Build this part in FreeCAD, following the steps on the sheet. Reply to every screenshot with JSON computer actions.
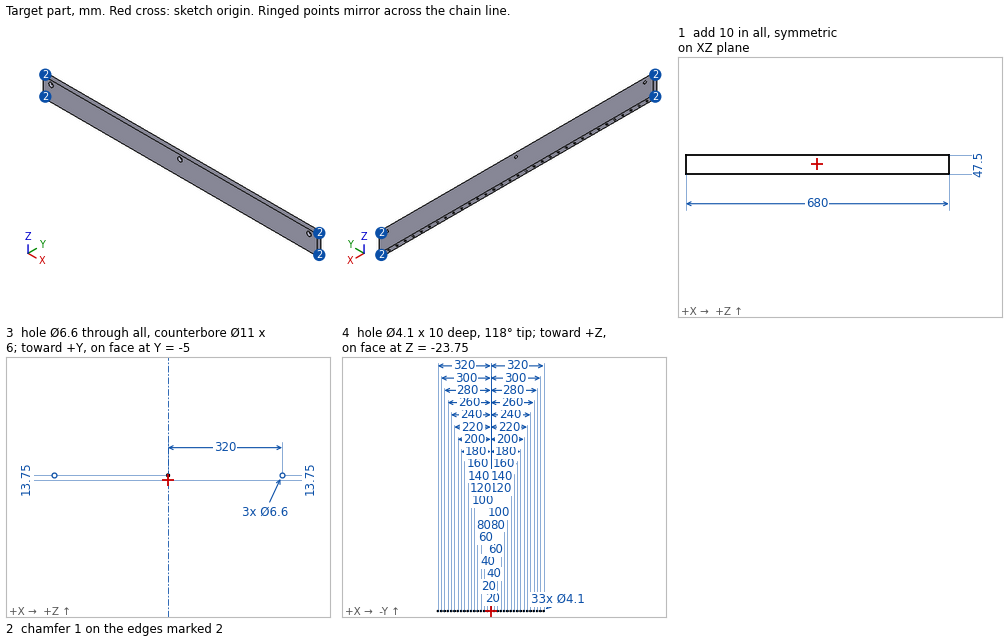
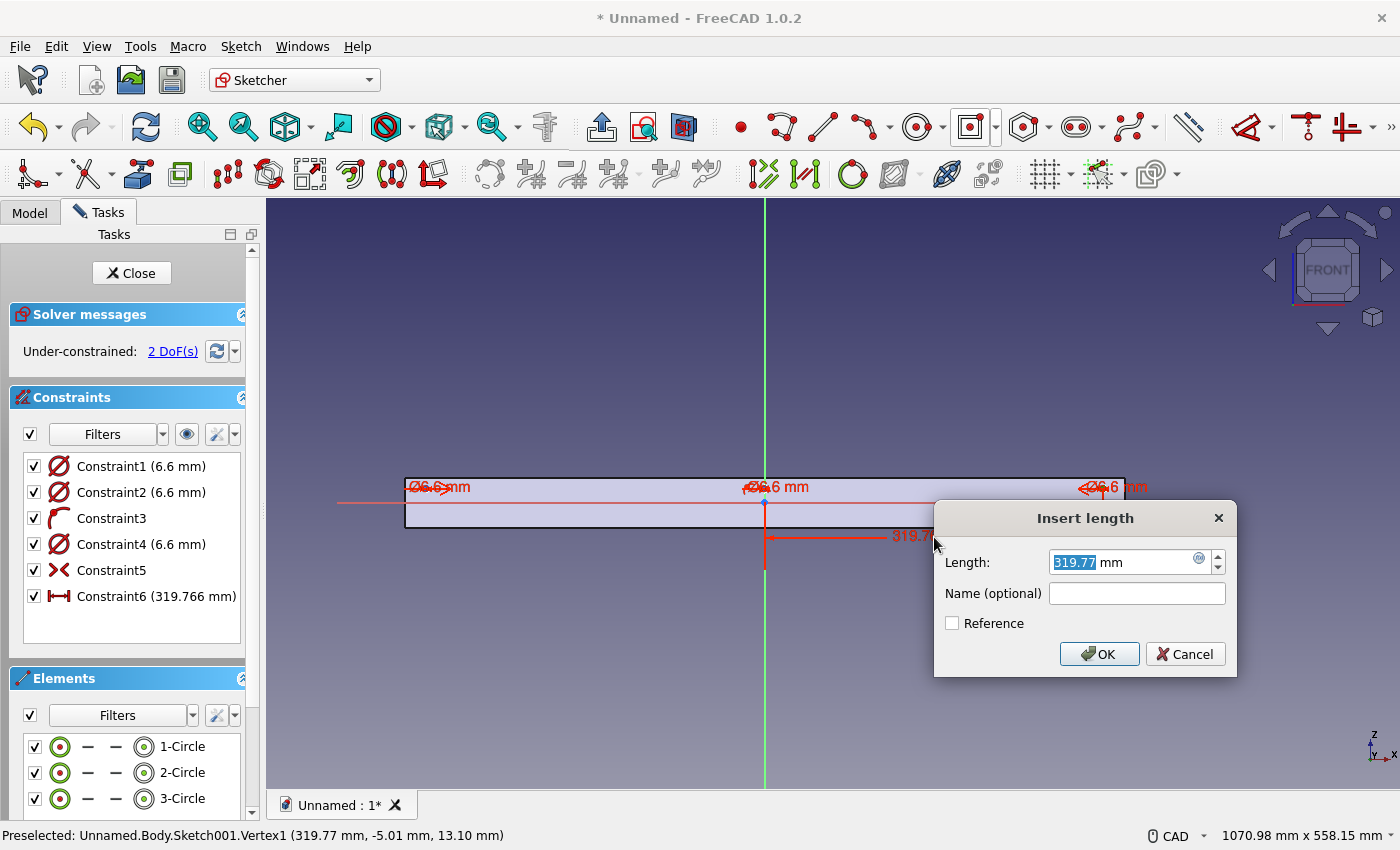
{"action": "type", "text": "320"}
{"action": "key", "text": "Return"}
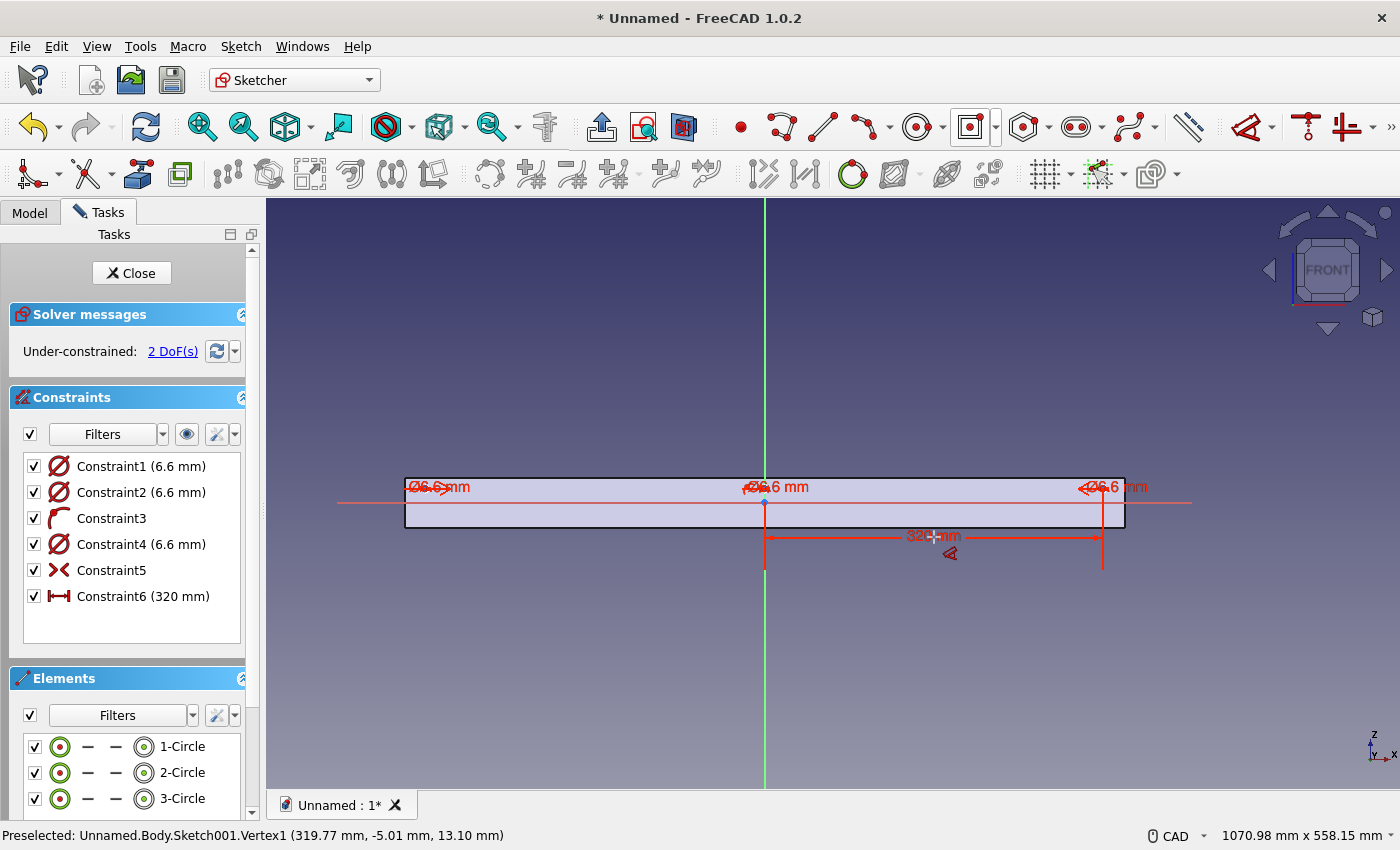
{"action": "scroll", "coordinate": [1103, 489], "scroll_direction": "up", "scroll_amount": 6}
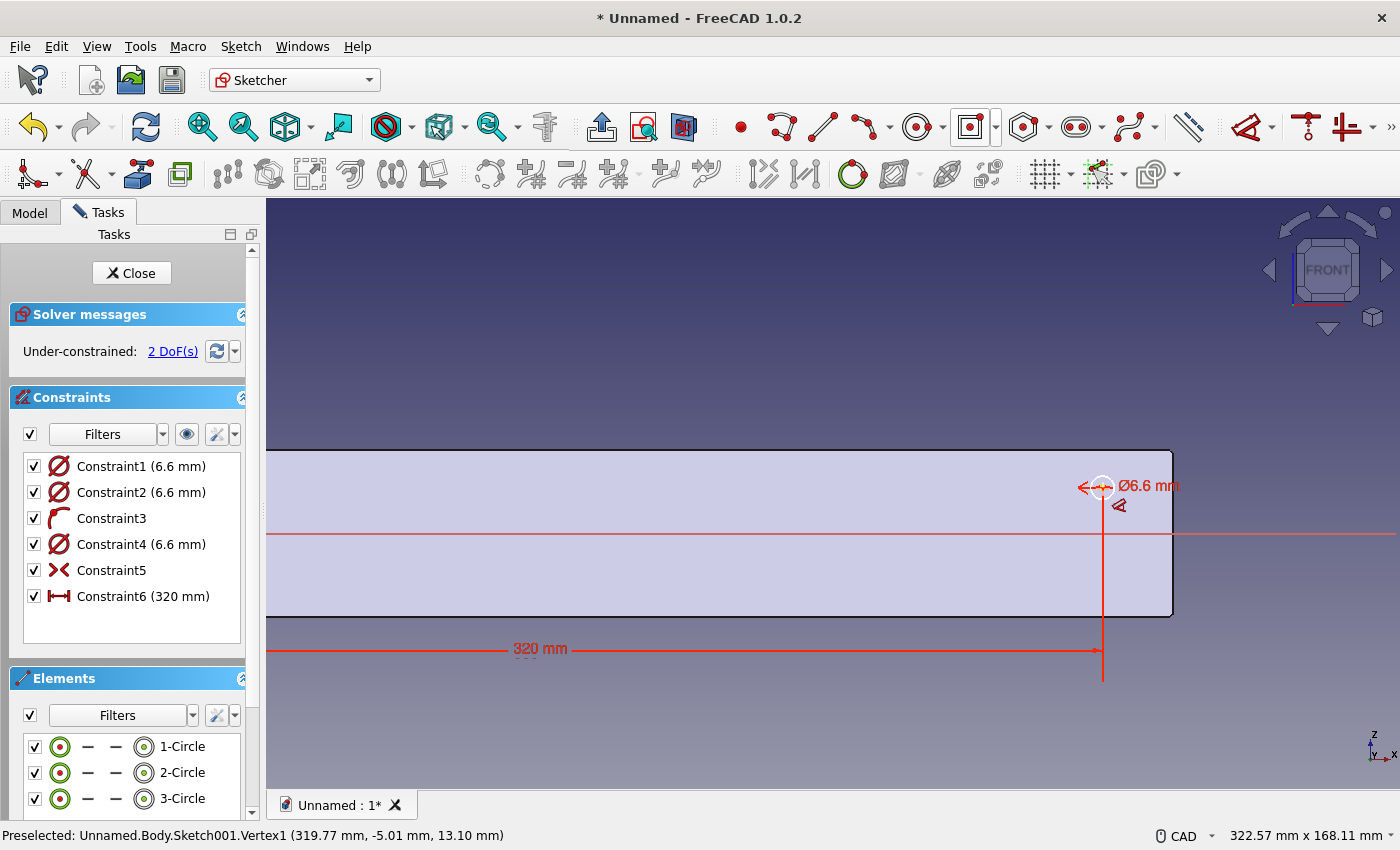
{"action": "left_click", "coordinate": [1103, 488]}
{"action": "left_click", "coordinate": [1137, 511]}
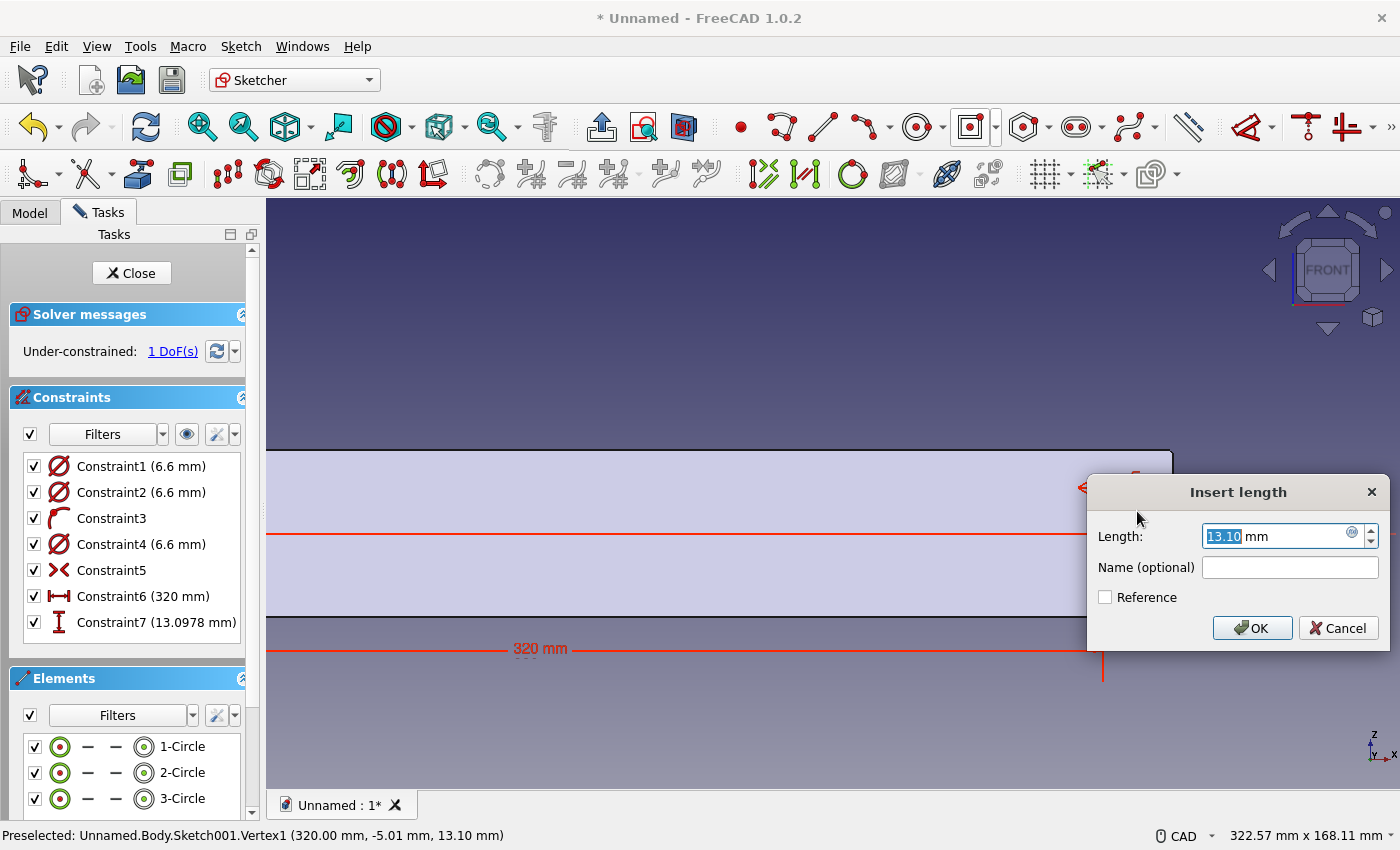
{"action": "type", "text": "13.75"}
{"action": "key", "text": "Return"}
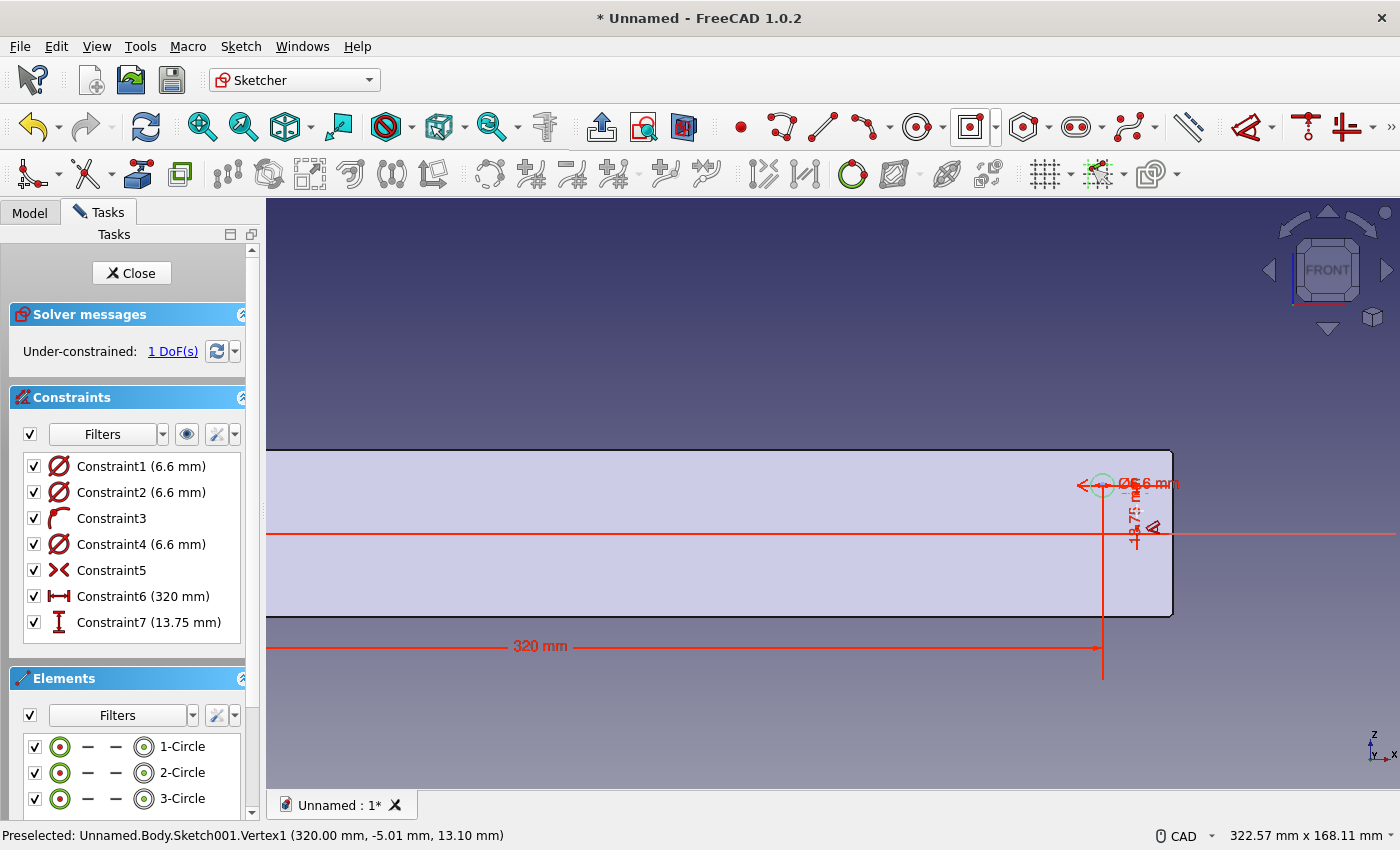
{"action": "scroll", "coordinate": [1104, 489], "scroll_direction": "down", "scroll_amount": 6}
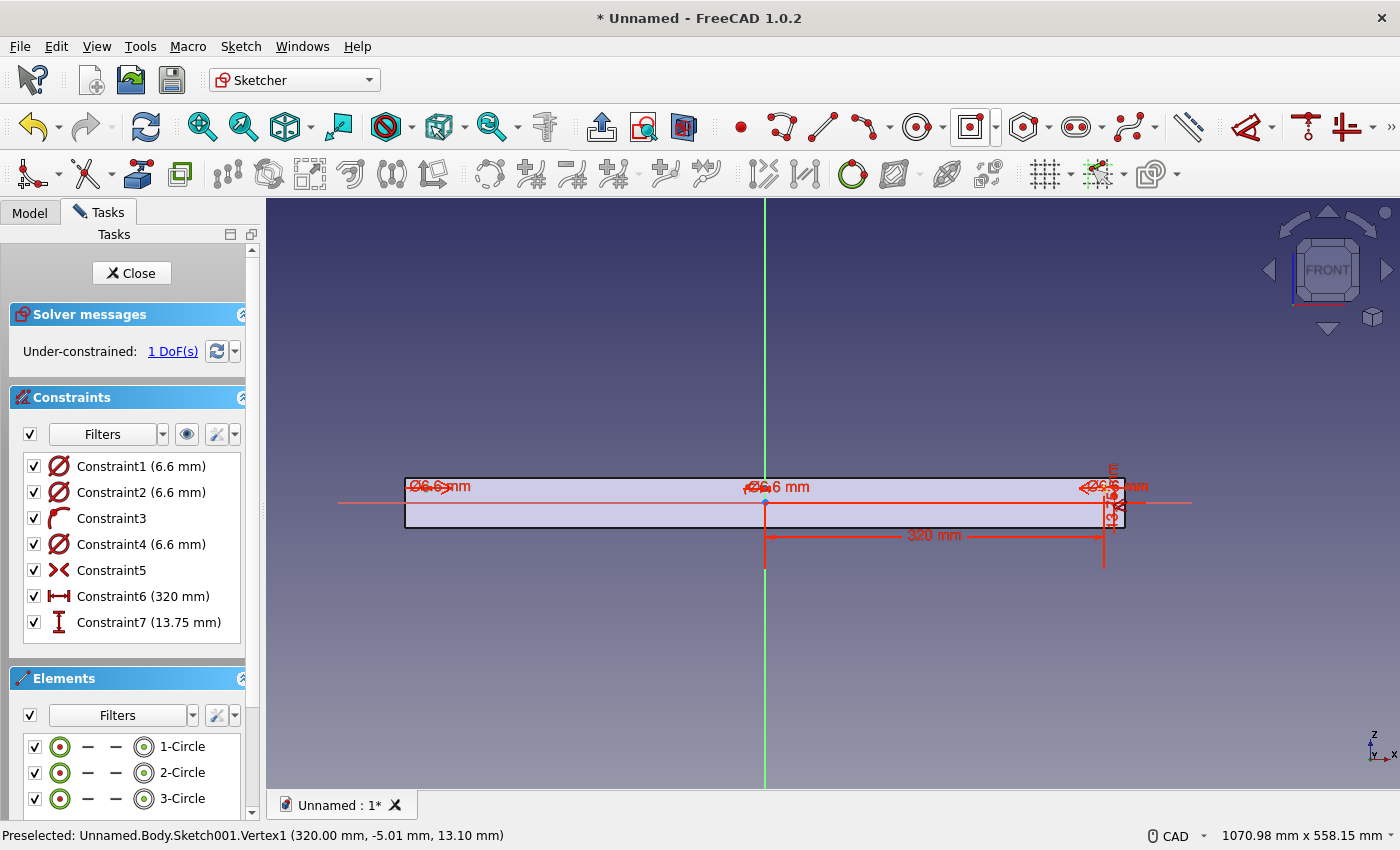
{"action": "scroll", "coordinate": [765, 489], "scroll_direction": "up", "scroll_amount": 6}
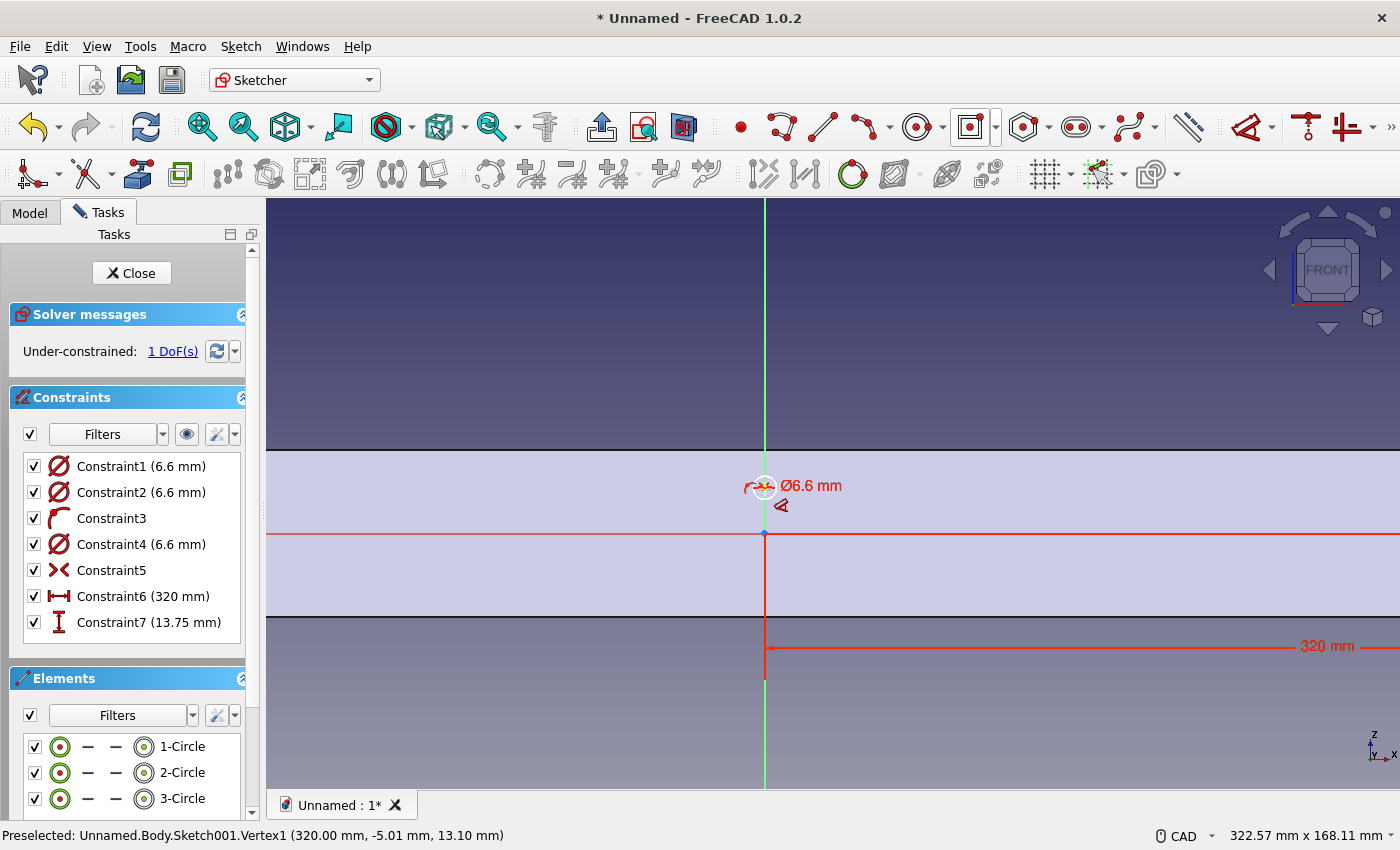
{"action": "left_click", "coordinate": [765, 488]}
{"action": "left_click", "coordinate": [799, 511]}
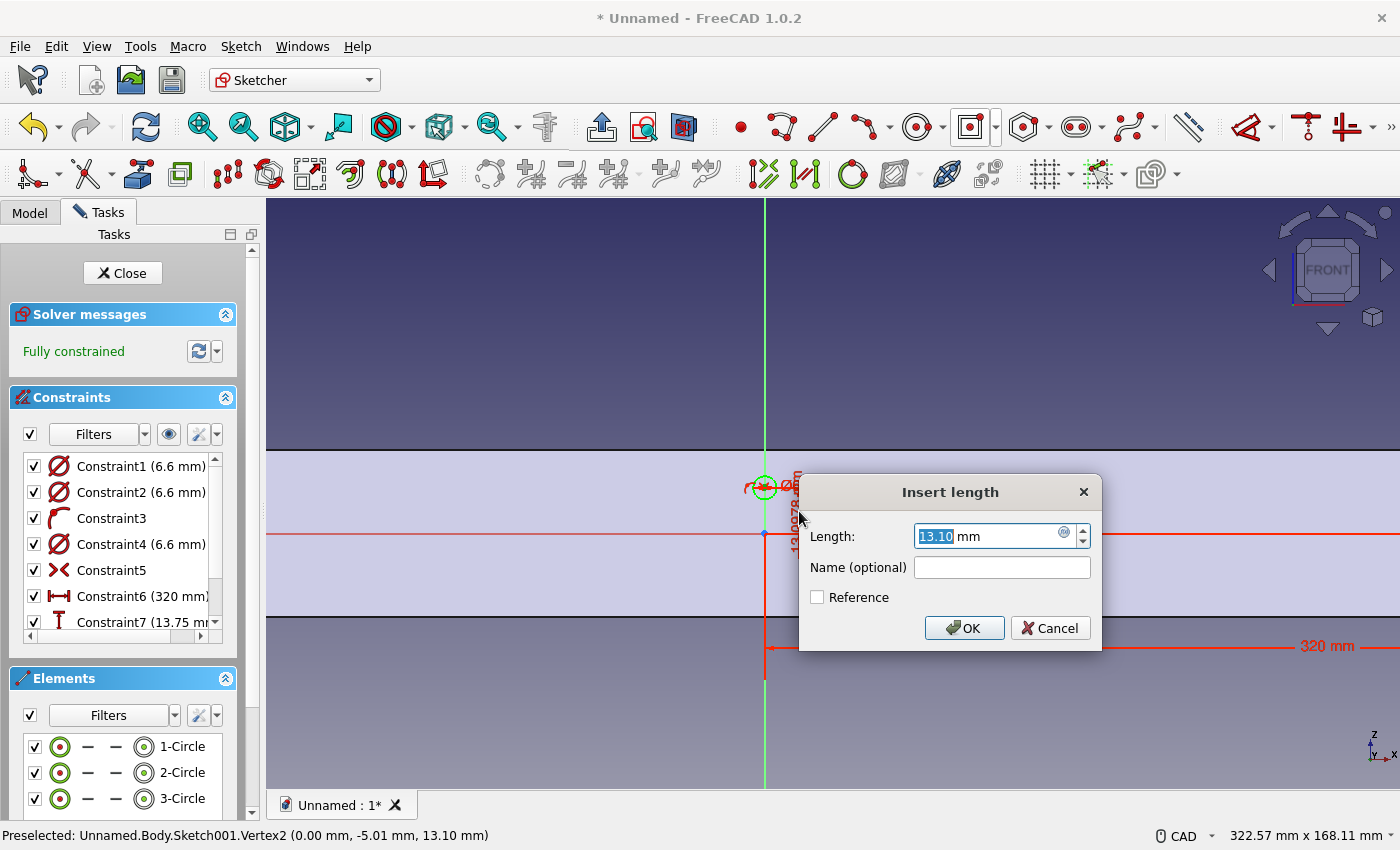
{"action": "type", "text": "13.75"}
{"action": "key", "text": "Return"}
{"action": "key", "text": "Escape"}